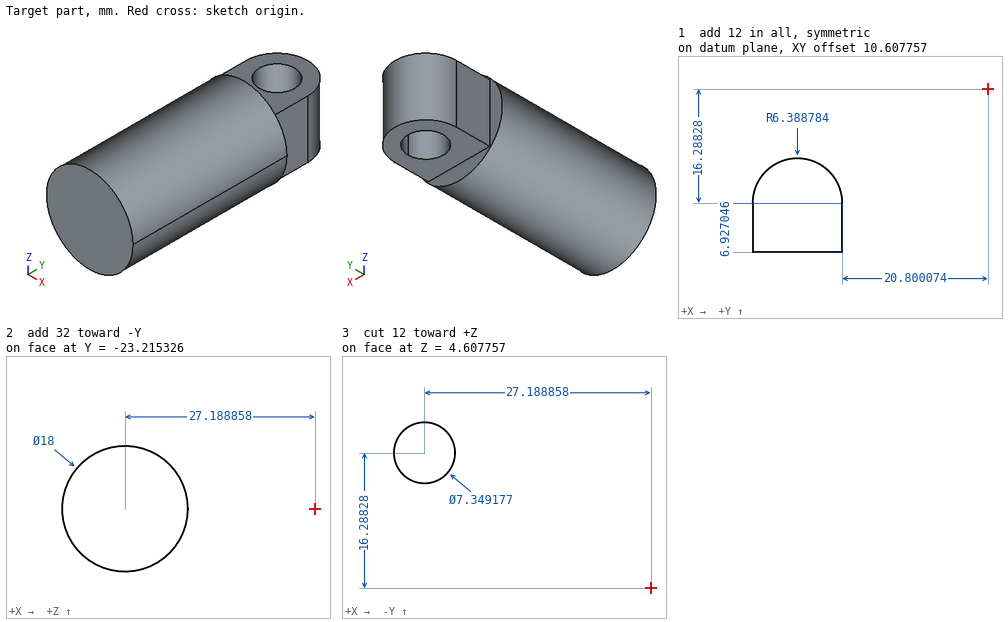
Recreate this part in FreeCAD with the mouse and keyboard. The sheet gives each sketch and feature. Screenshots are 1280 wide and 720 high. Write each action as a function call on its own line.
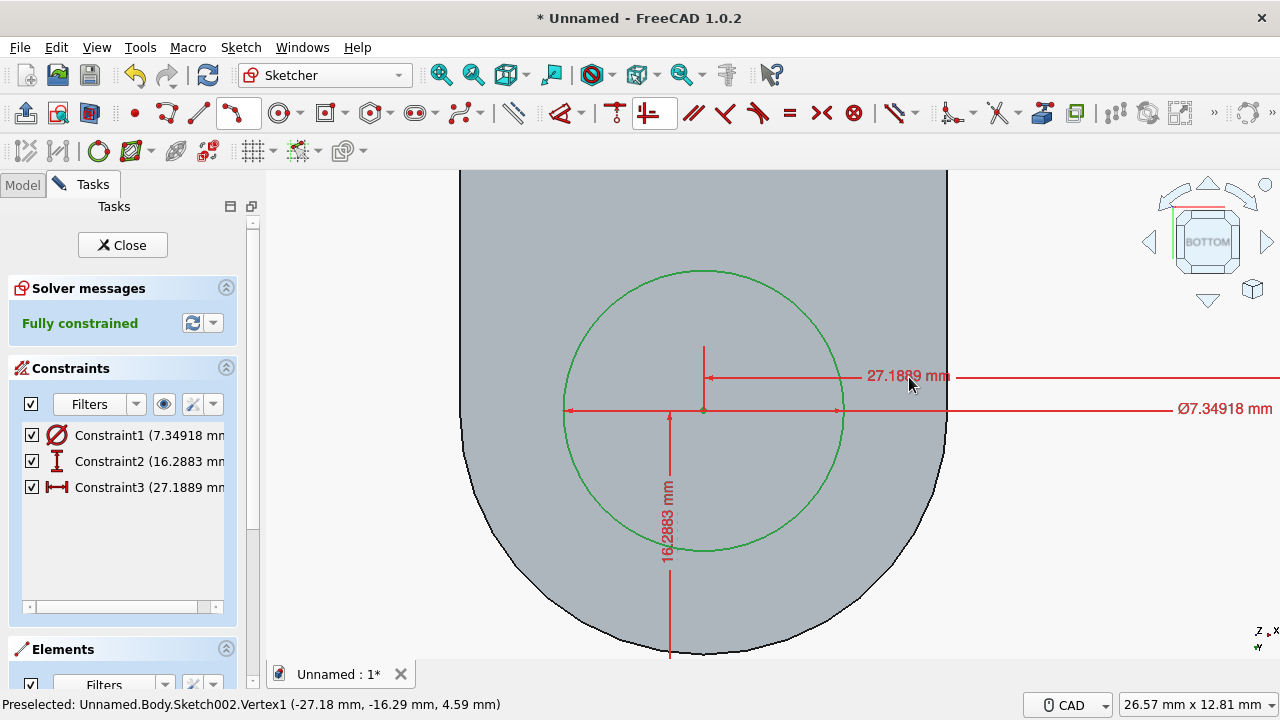
click(123, 245)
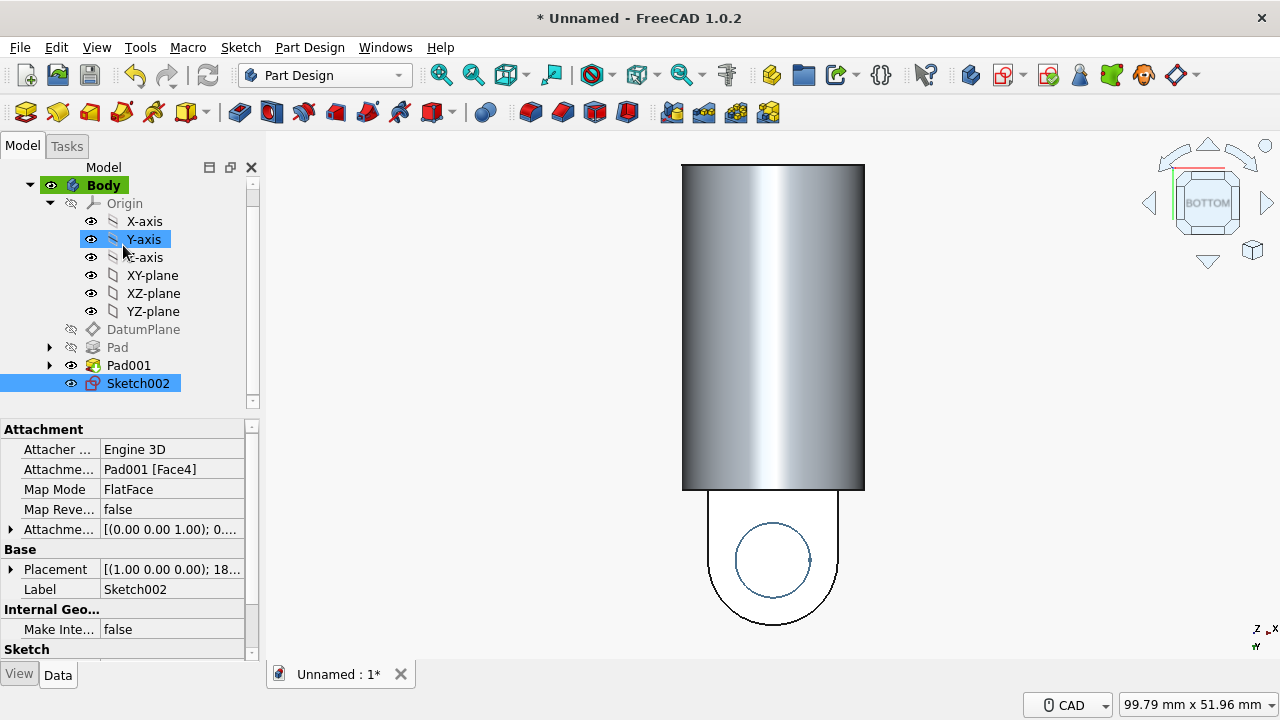
click(240, 112)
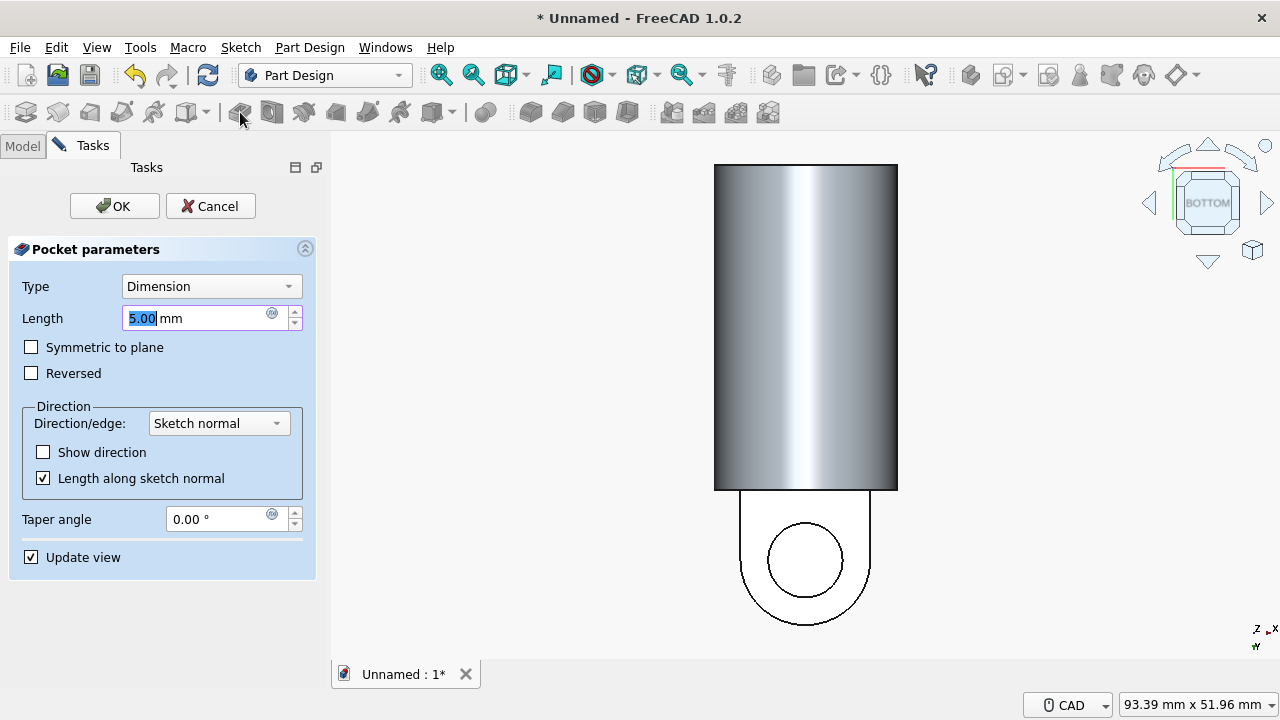
text(12)
key(Tab)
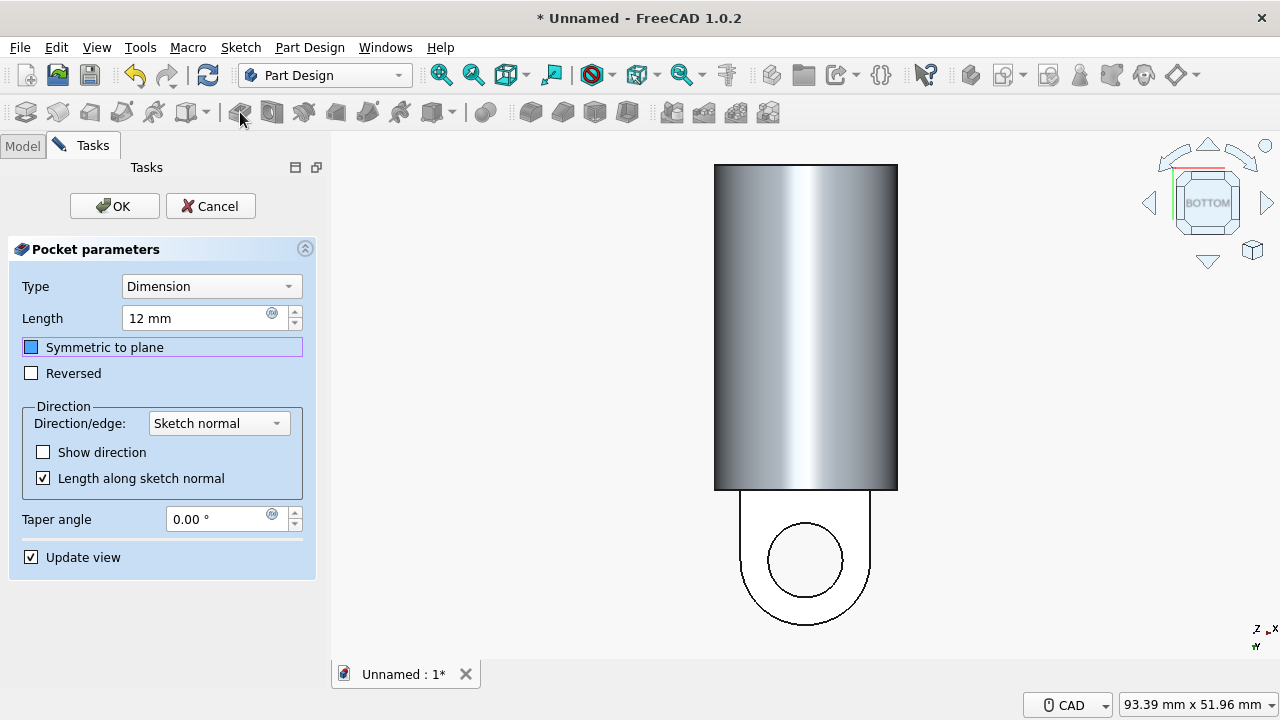
click(115, 206)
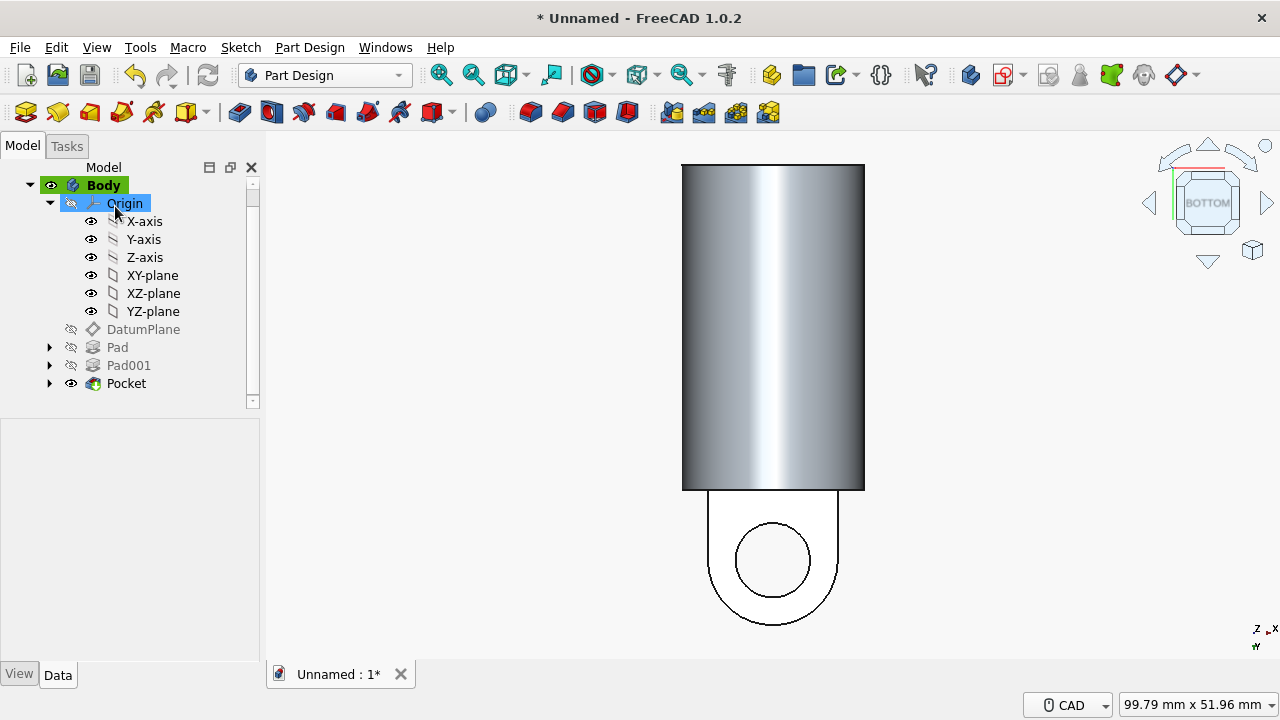
key(0)